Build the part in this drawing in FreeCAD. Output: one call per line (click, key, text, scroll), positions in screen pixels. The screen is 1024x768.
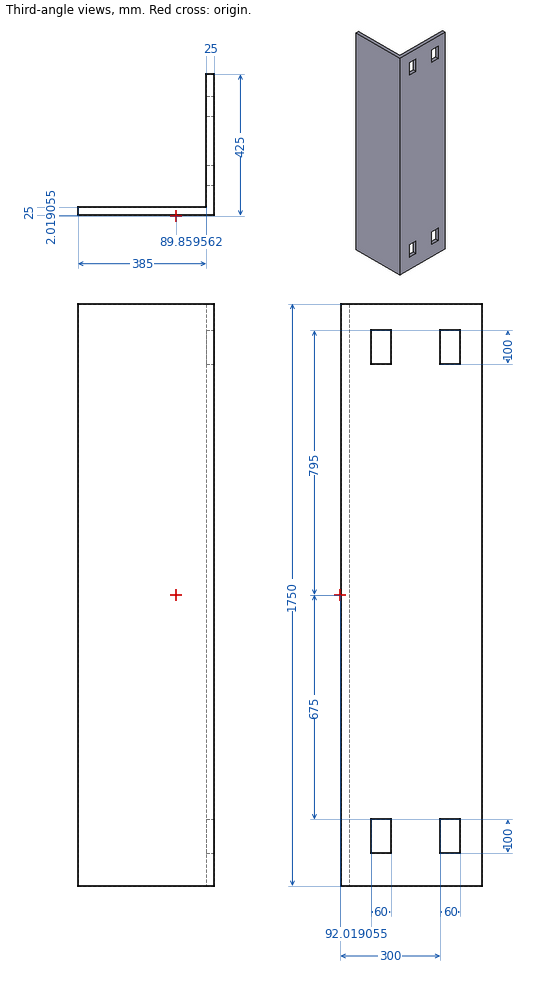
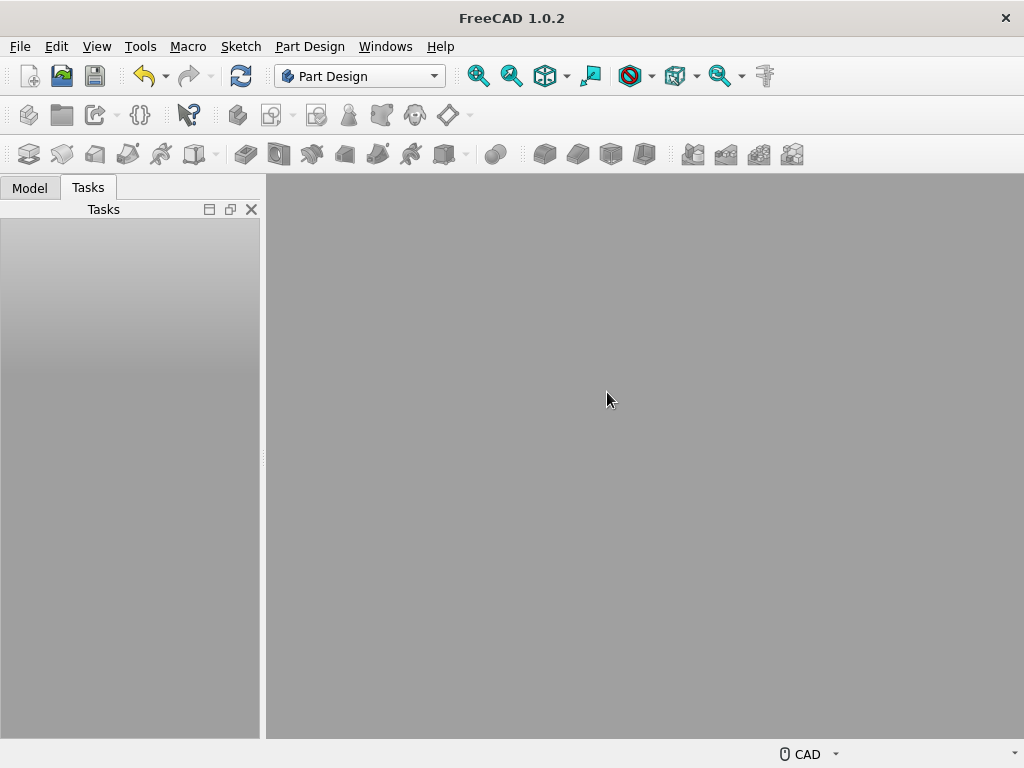
click(29, 76)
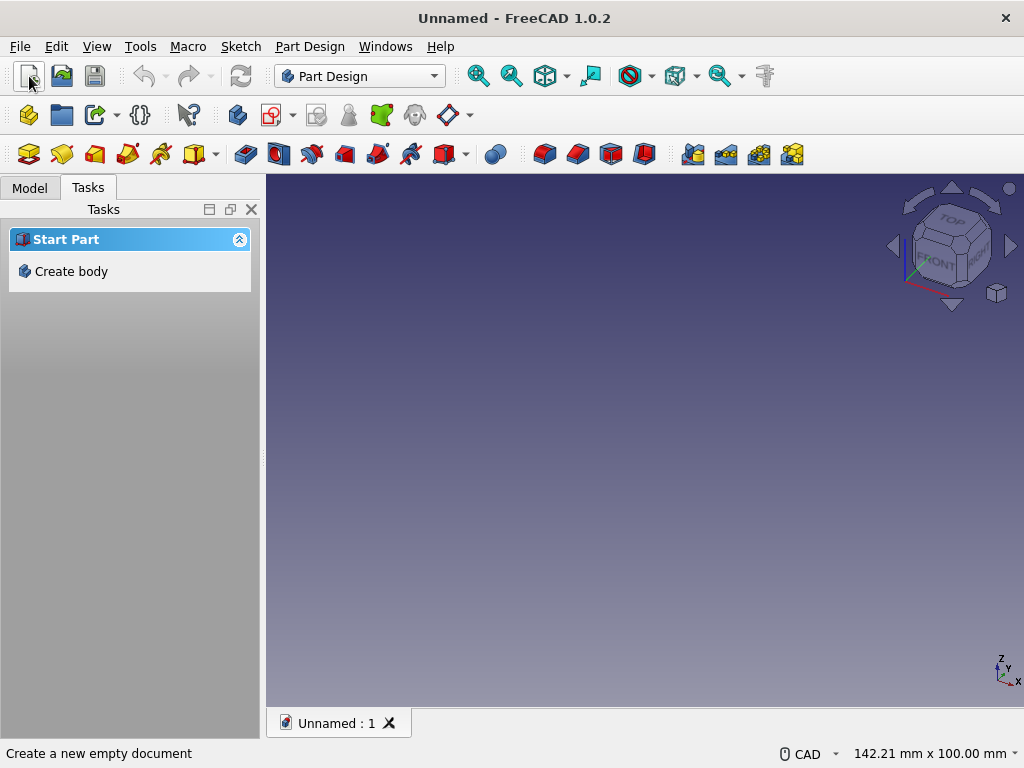
click(270, 116)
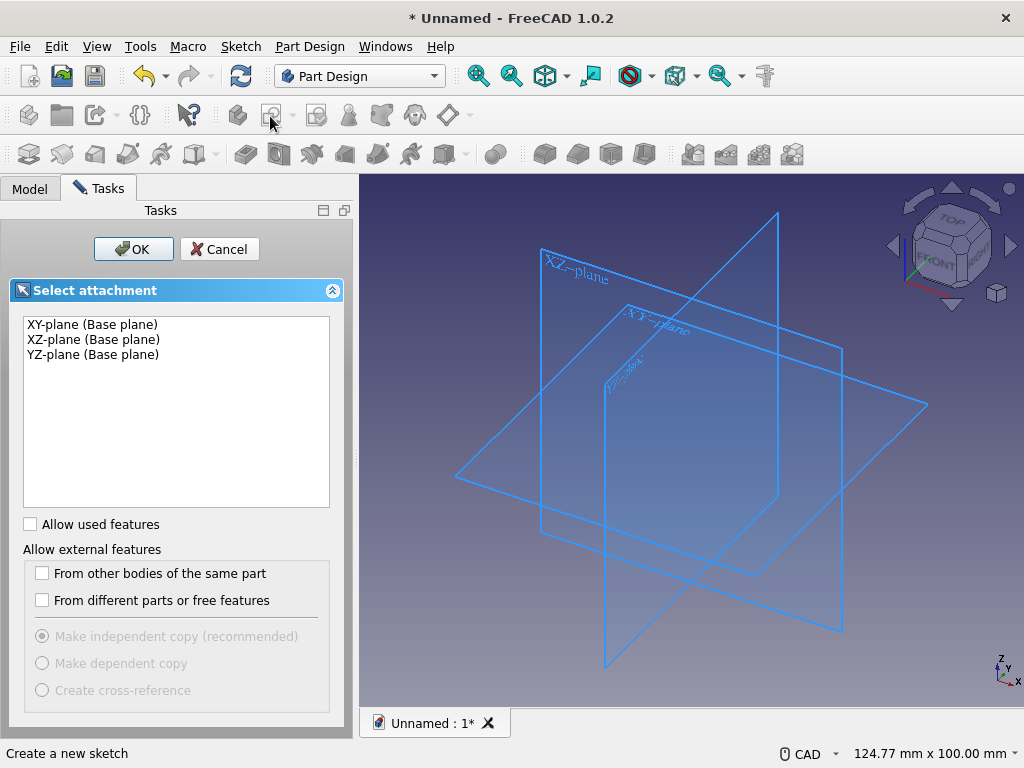
click(84, 324)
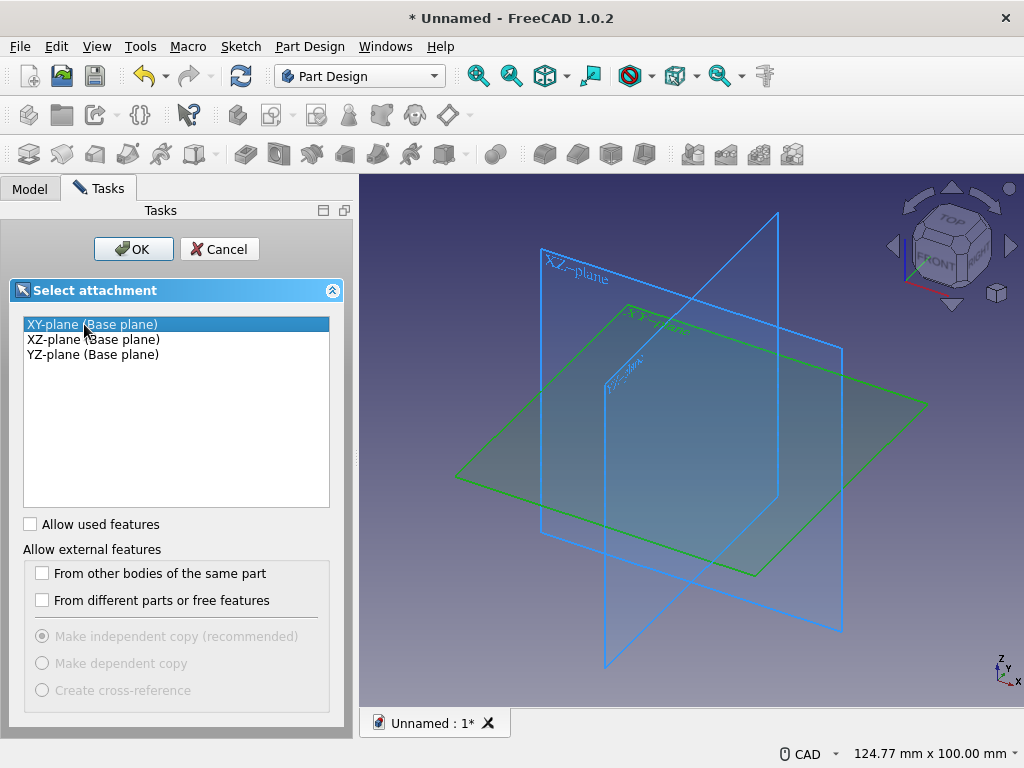
click(134, 249)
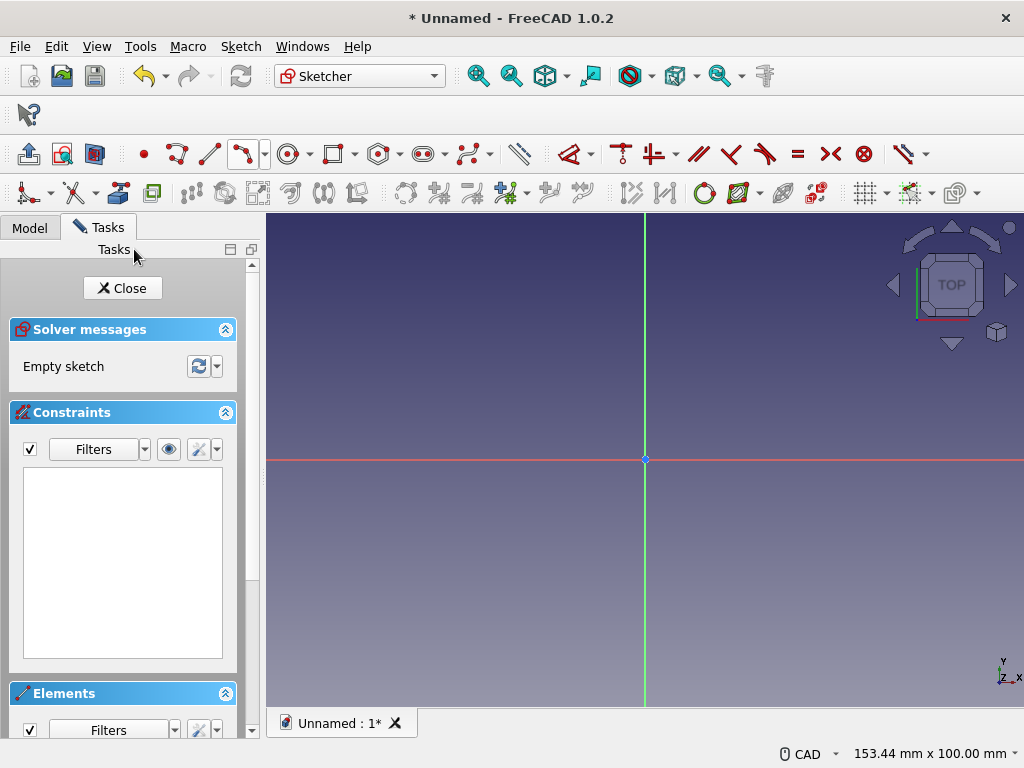
scroll(635, 624, down, 10)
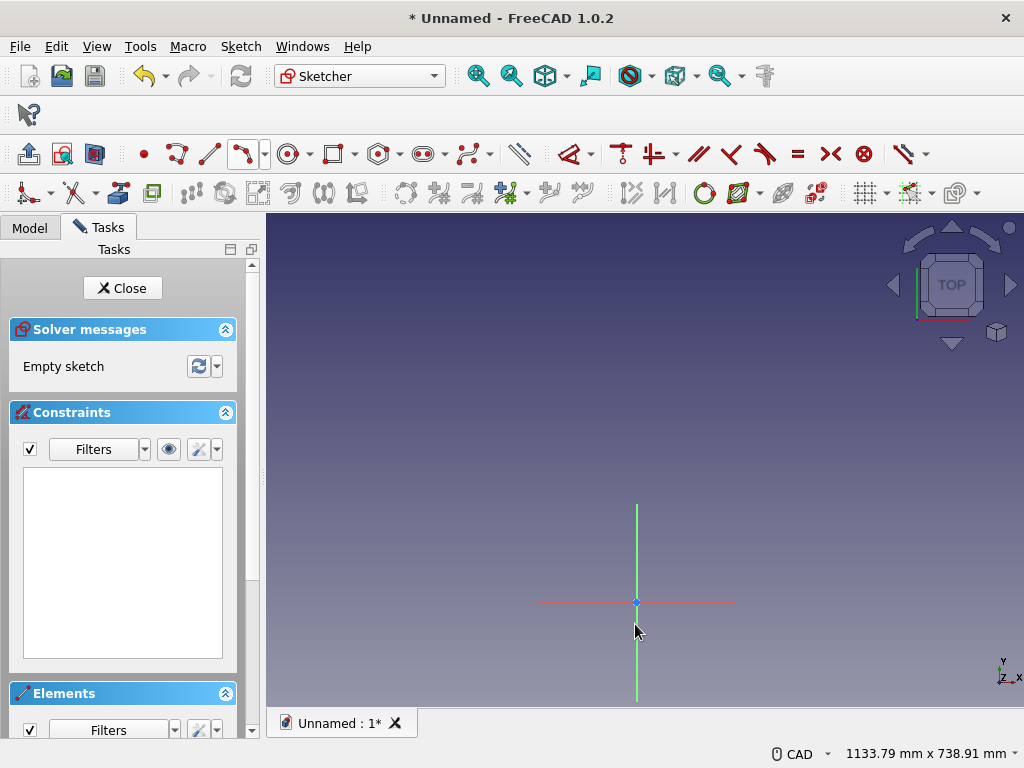
click(177, 154)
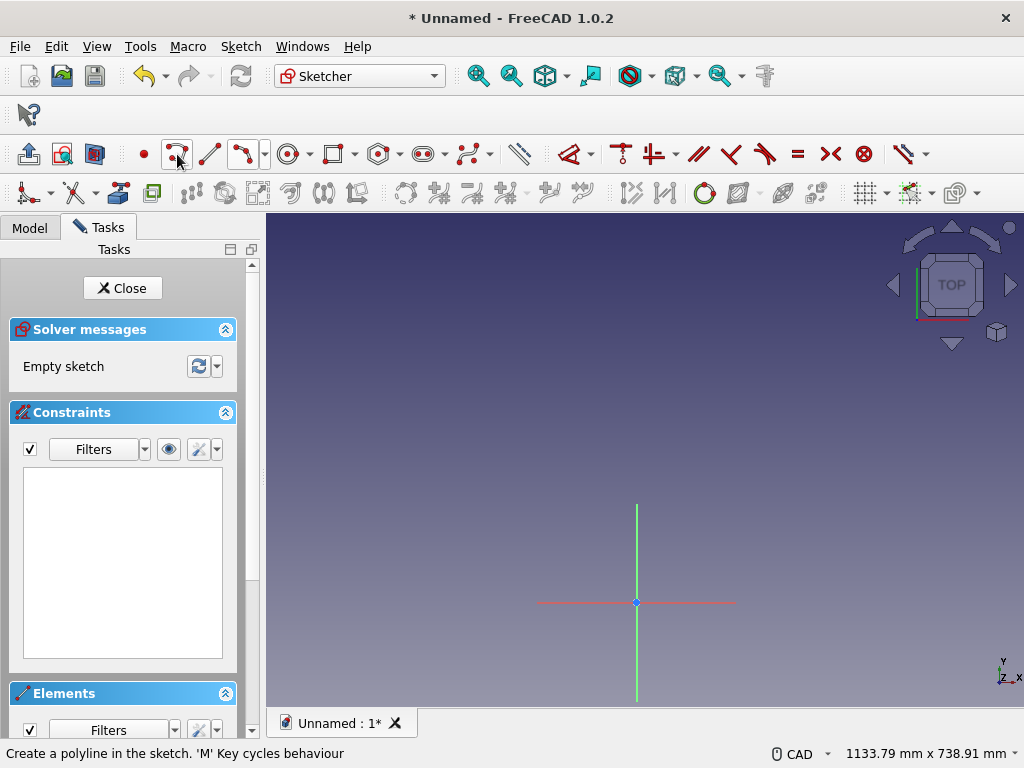
click(697, 584)
click(439, 584)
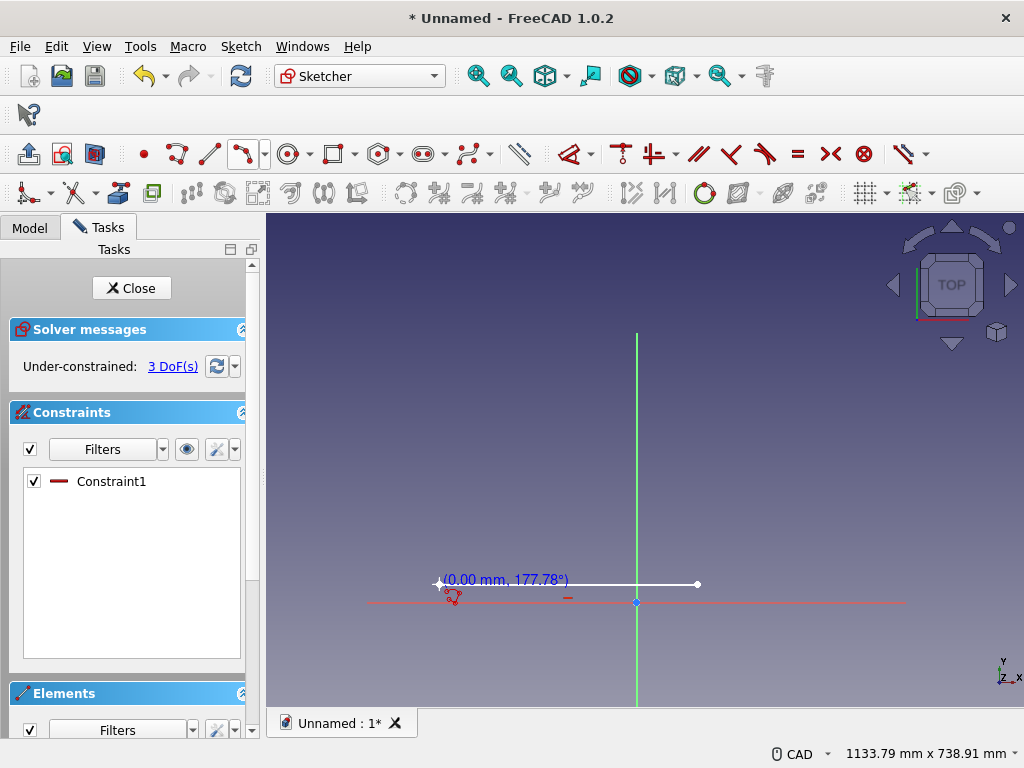
scroll(439, 601, up, 13)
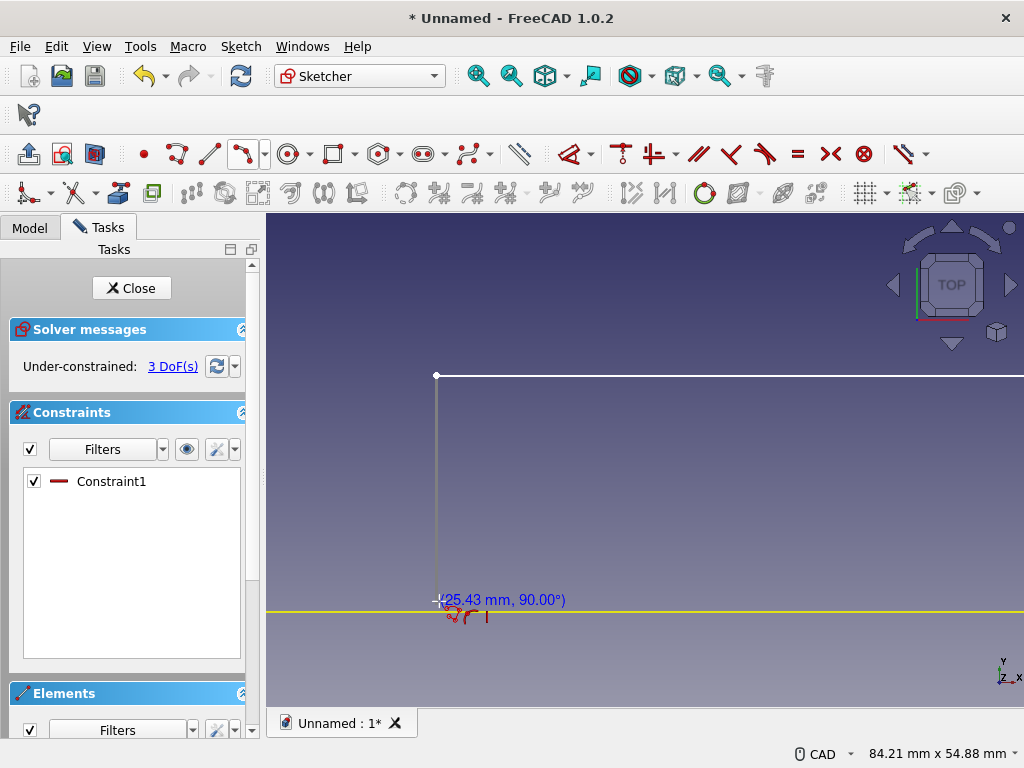
click(436, 594)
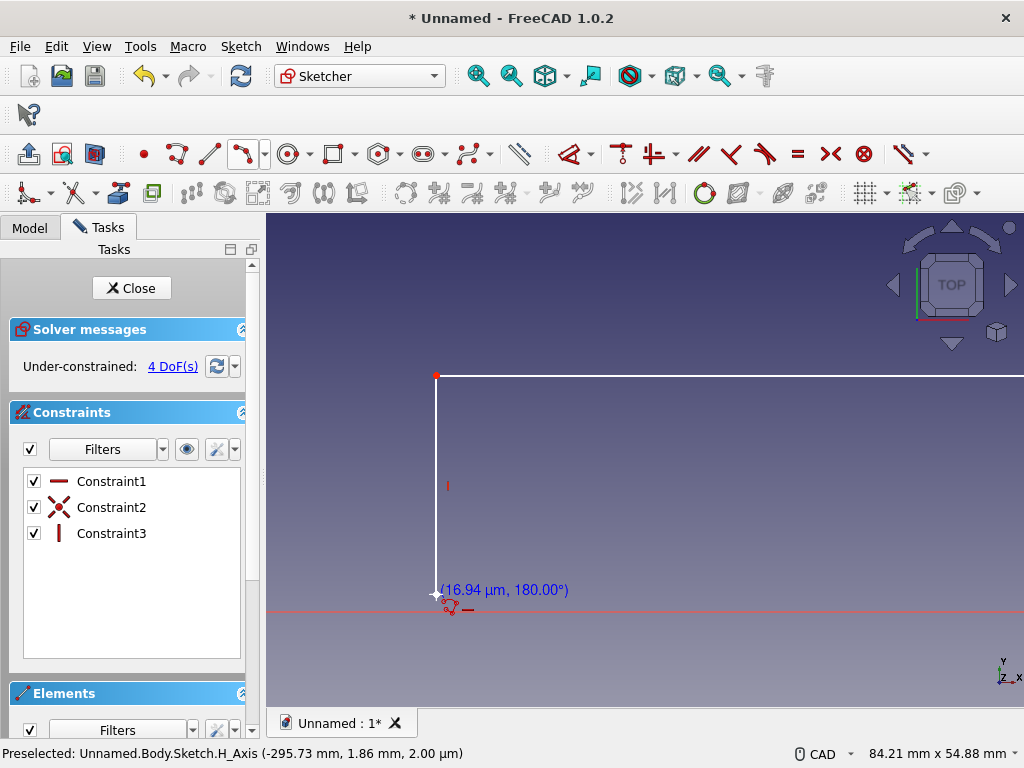
scroll(439, 601, down, 13)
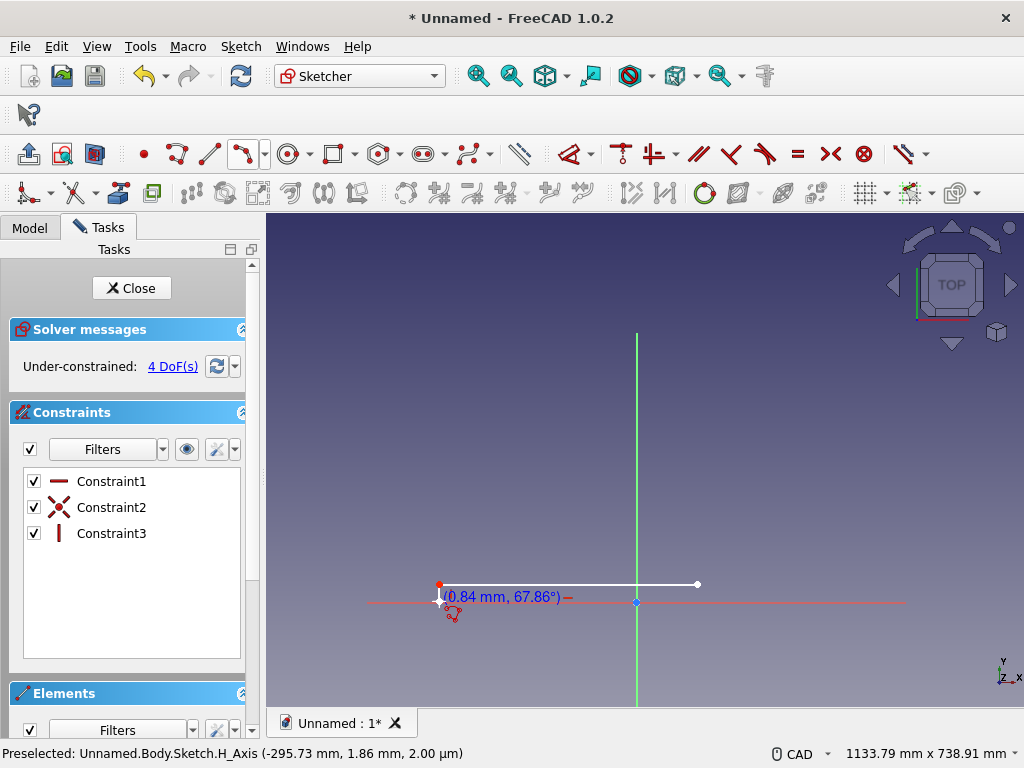
scroll(714, 601, up, 13)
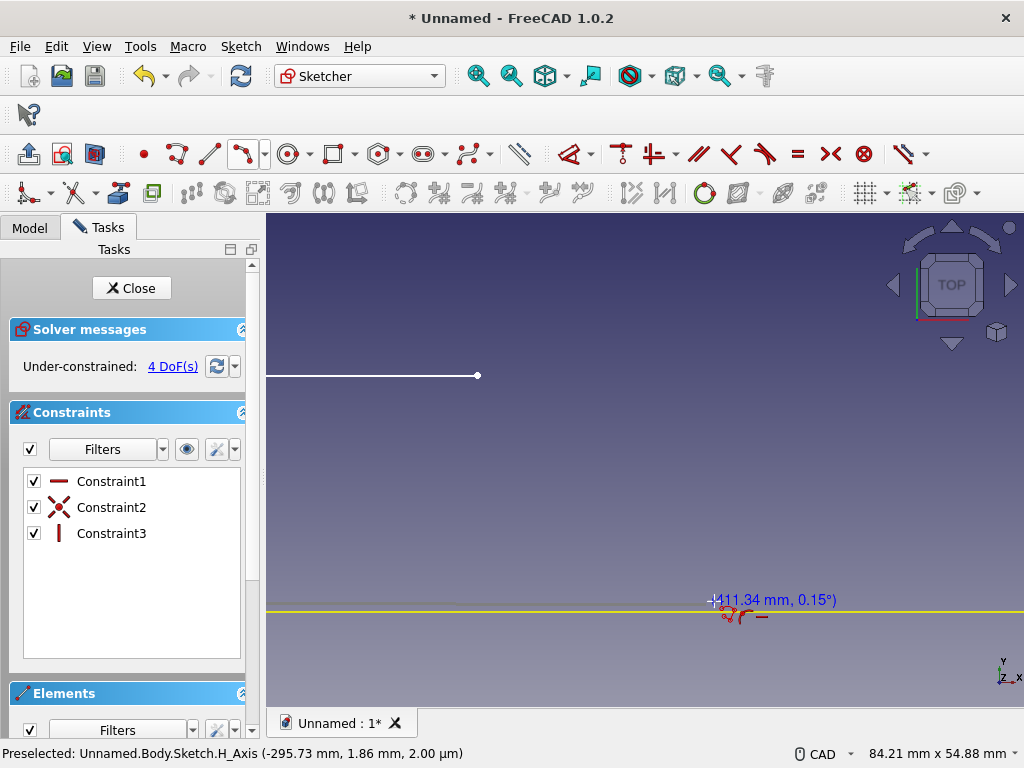
click(701, 594)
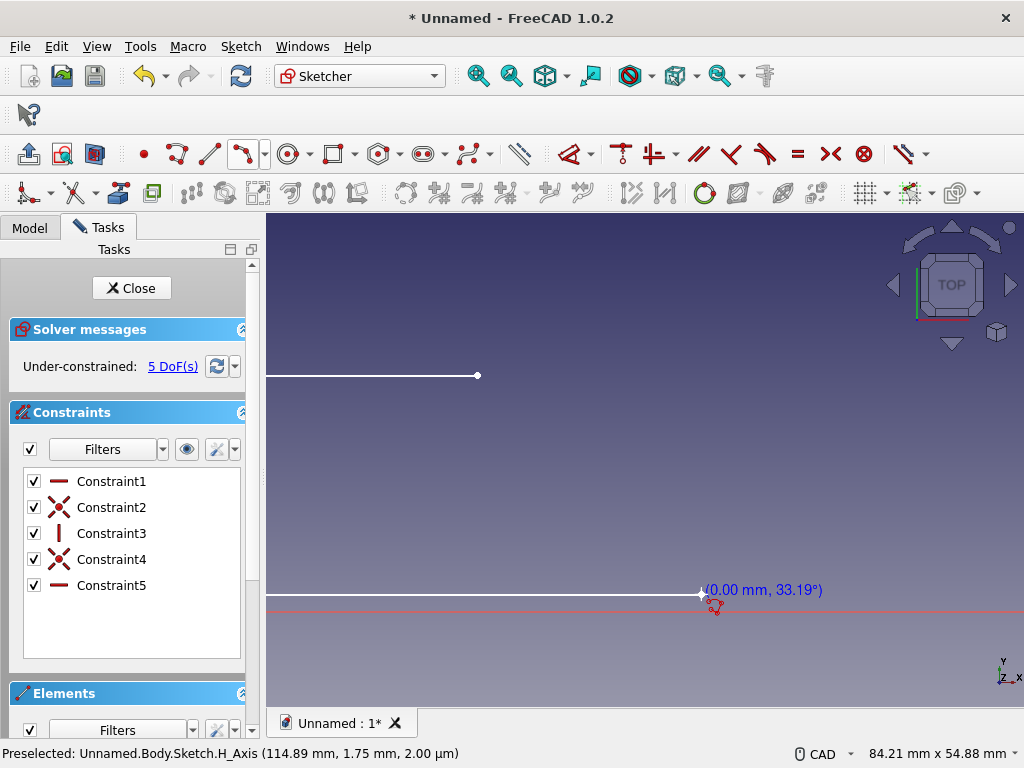
scroll(715, 601, down, 13)